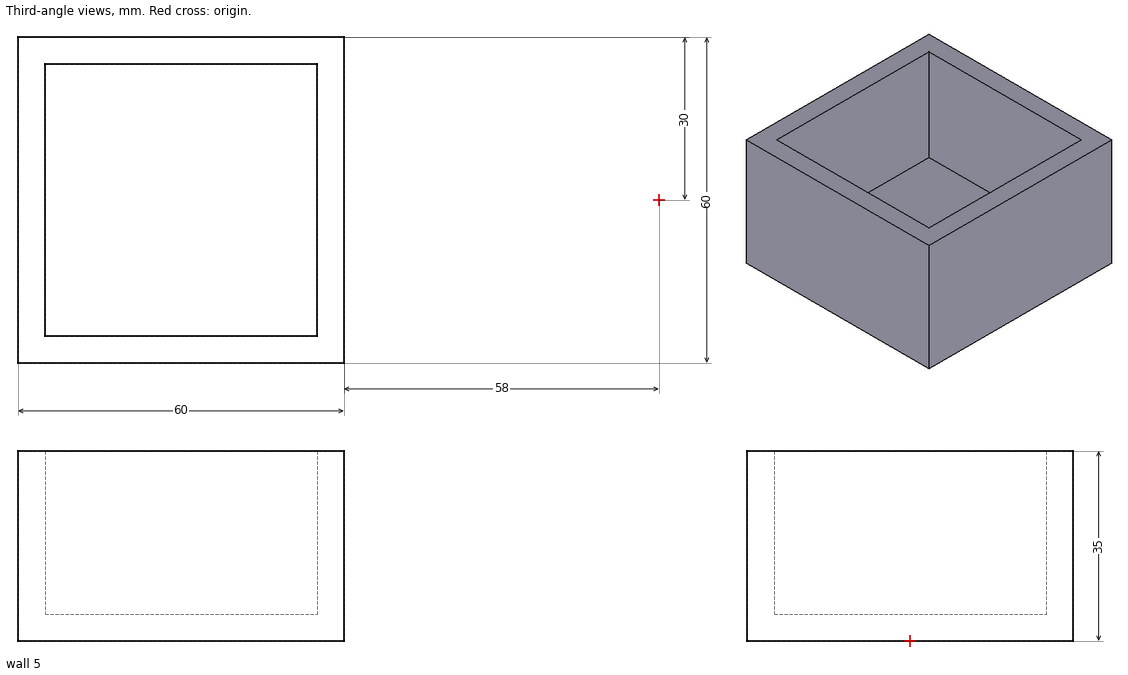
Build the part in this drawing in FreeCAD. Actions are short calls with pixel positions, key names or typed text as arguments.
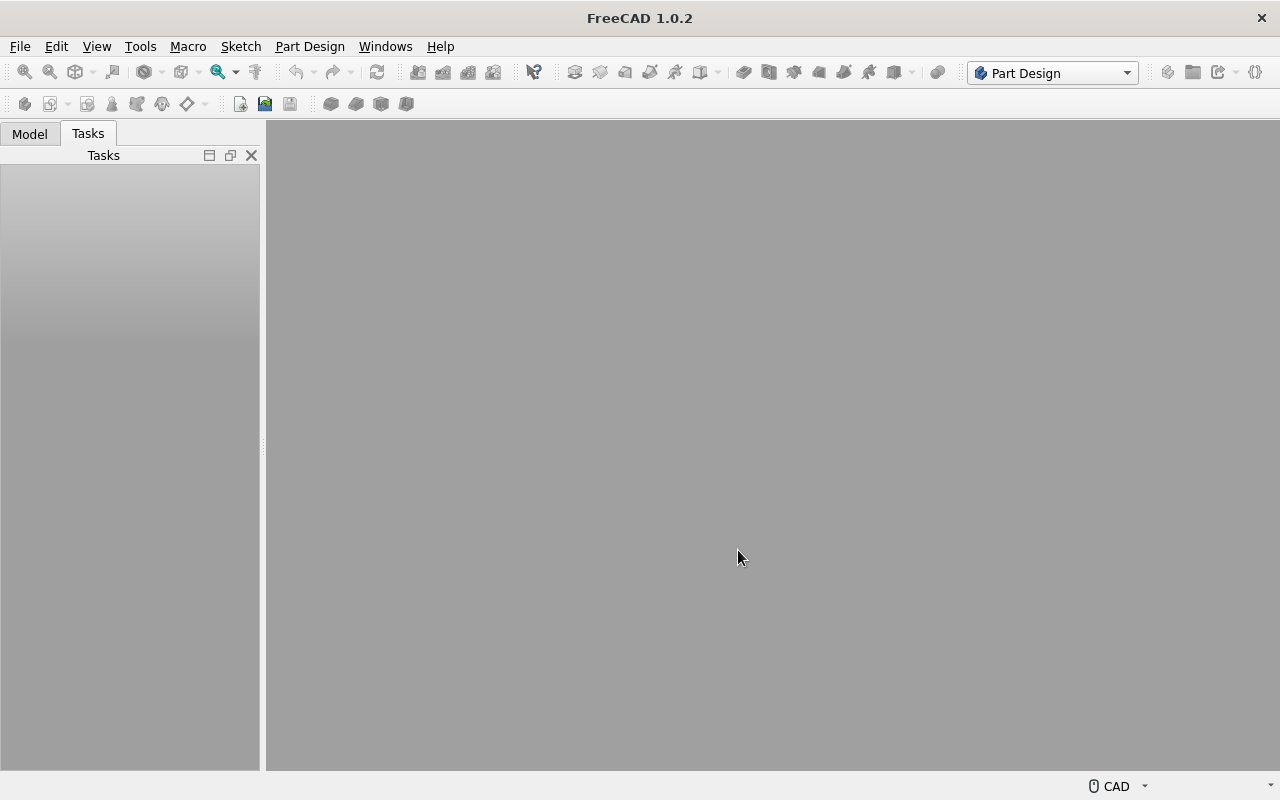
key(ctrl+n)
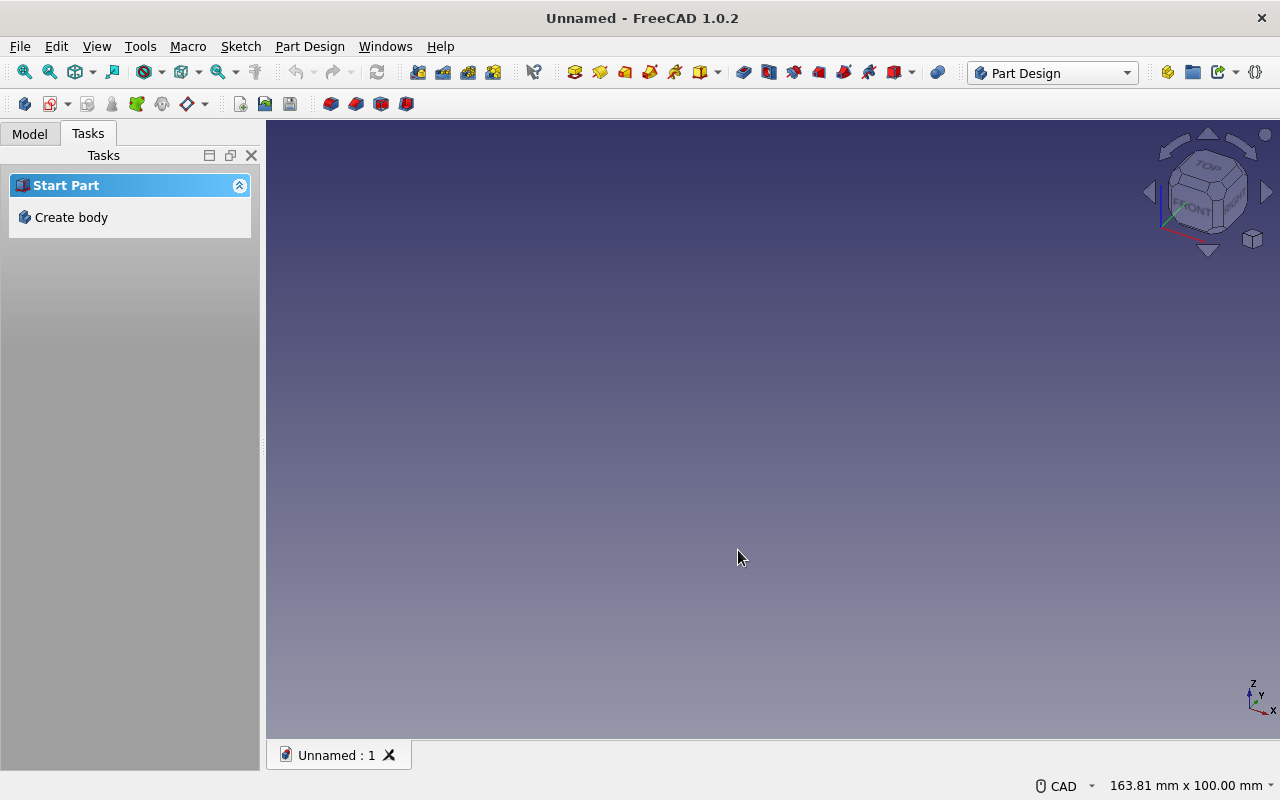
click(50, 104)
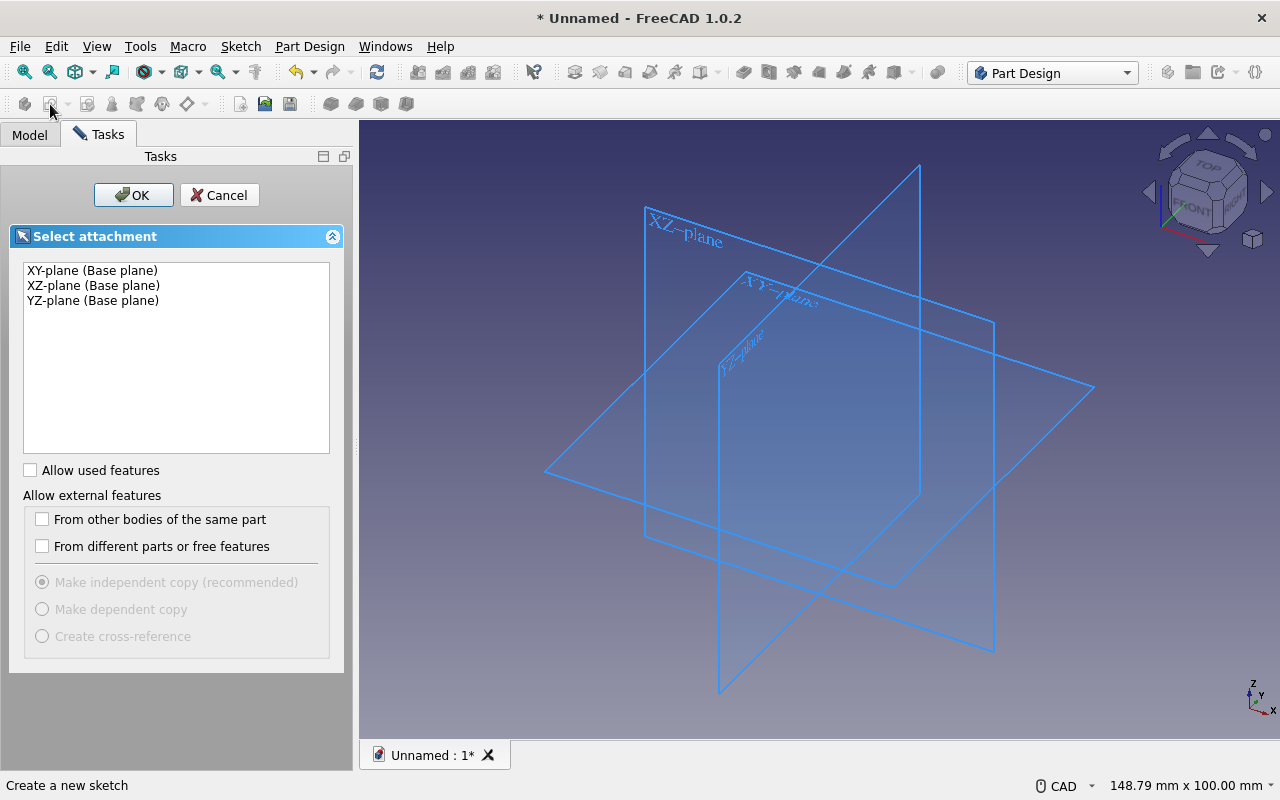
click(84, 270)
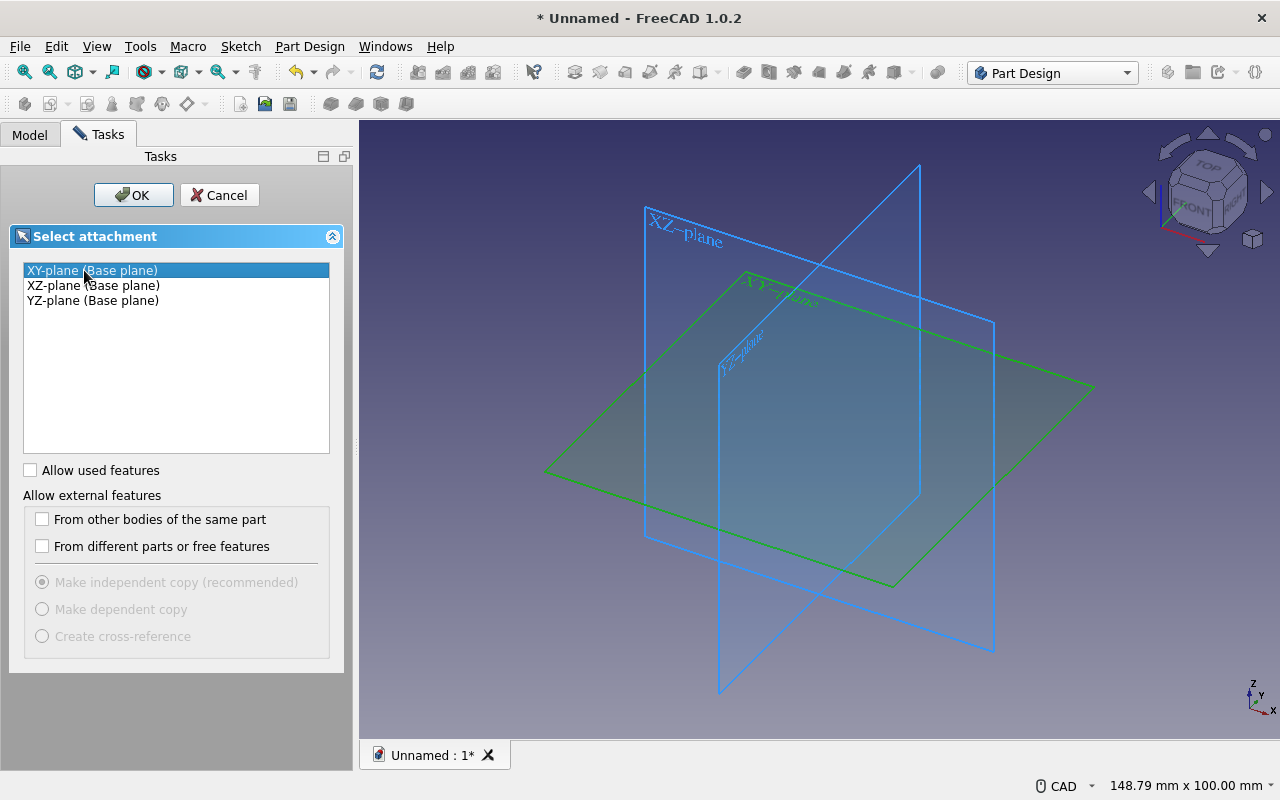
click(134, 195)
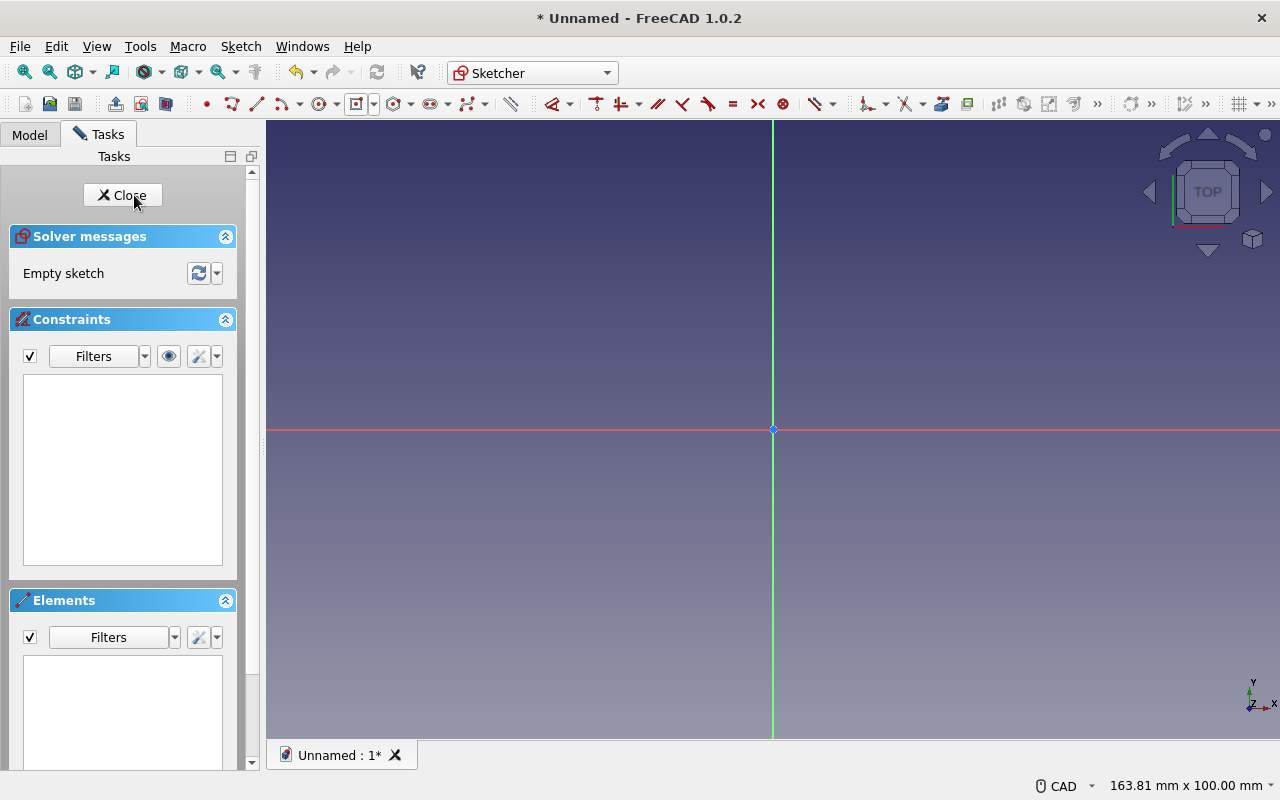
scroll(1115, 429, down, 2)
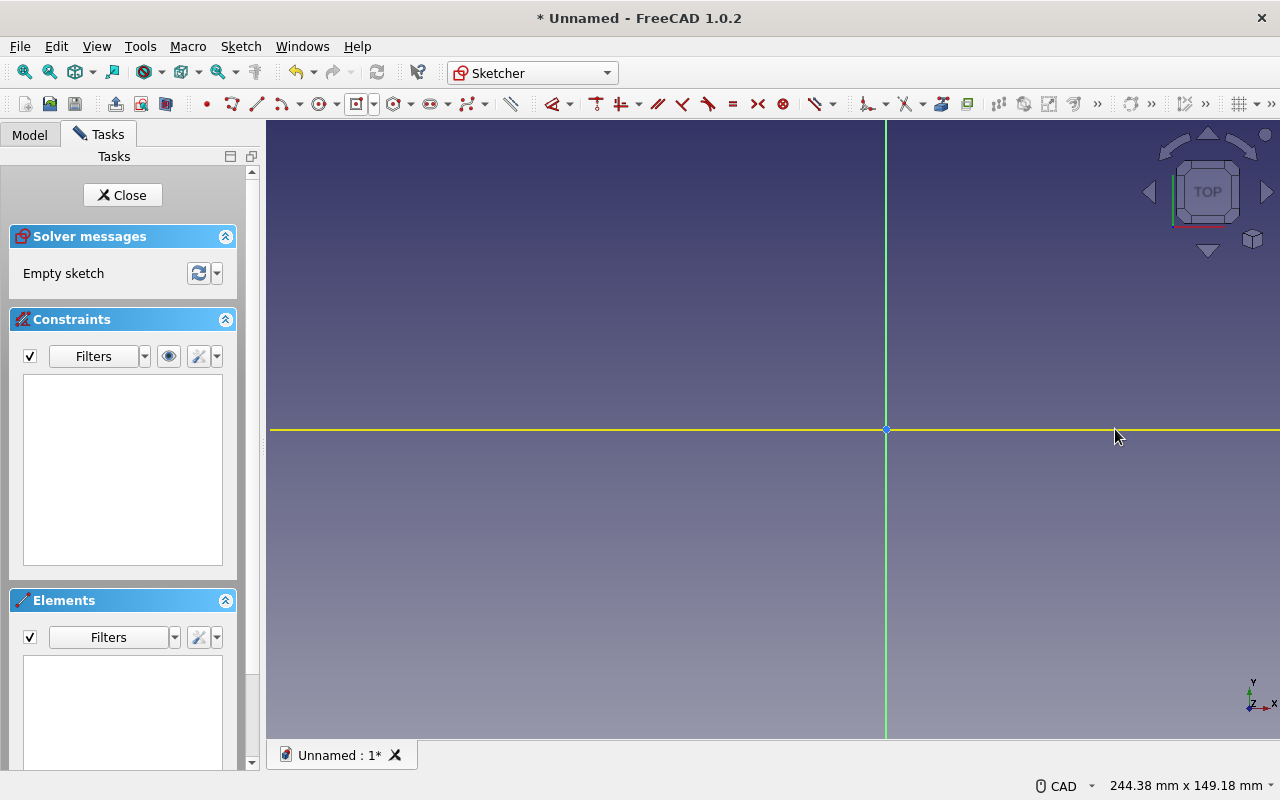
key(g)
key(r)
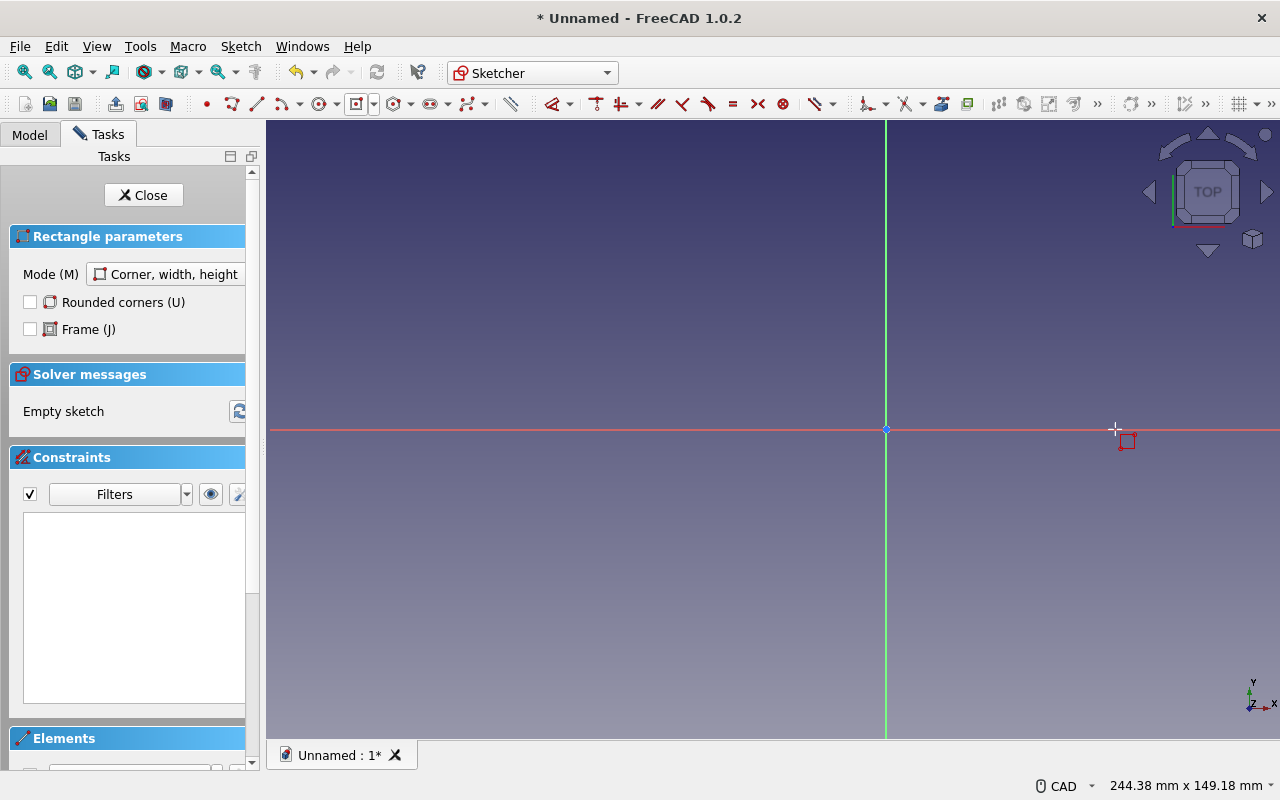
click(396, 305)
move(645, 554)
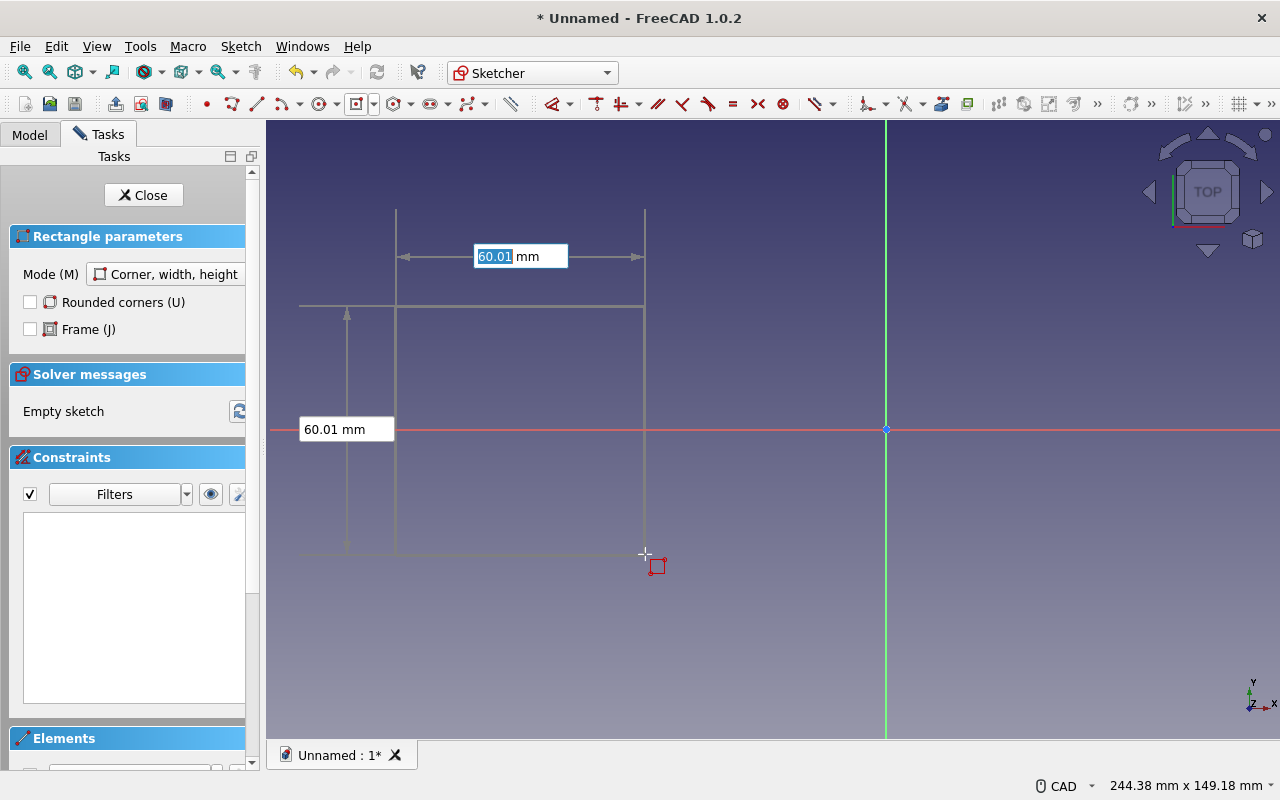
text(60)
key(Tab)
text(60)
key(Return)
key(Escape)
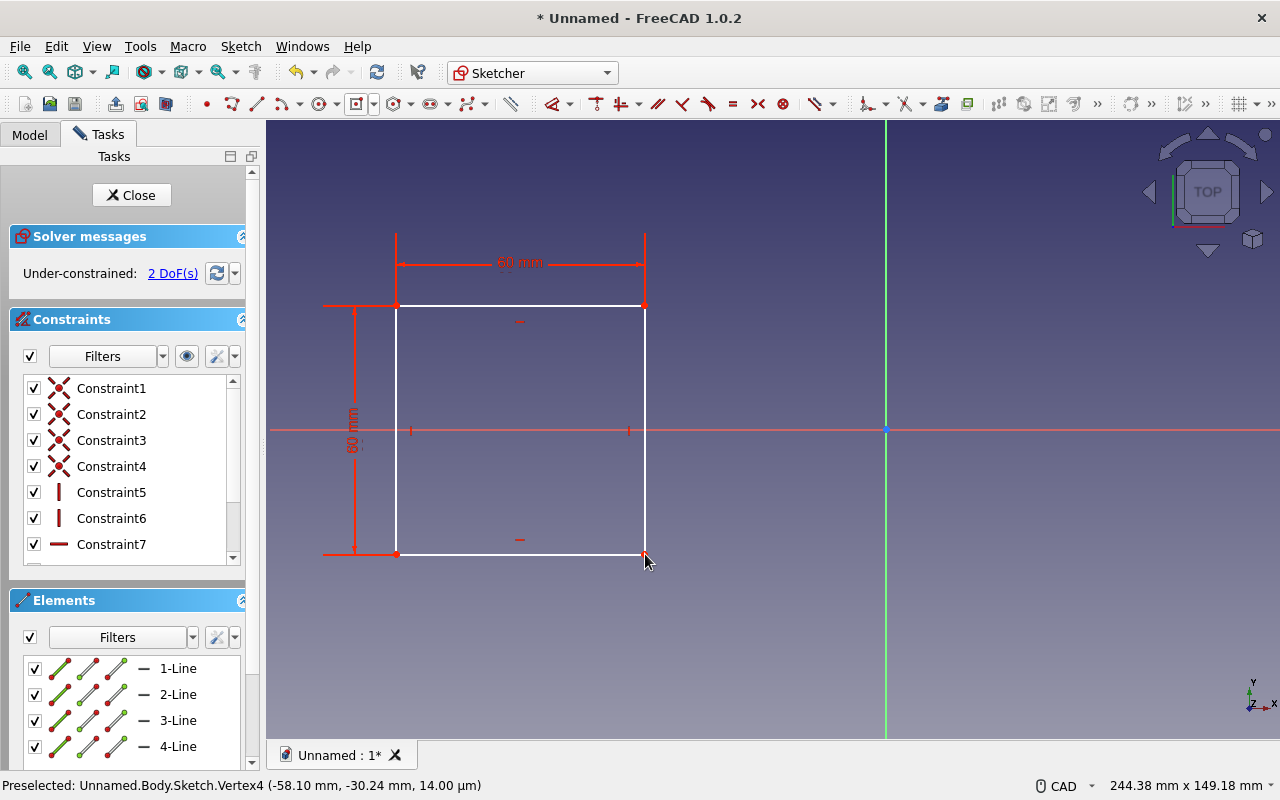
key(d)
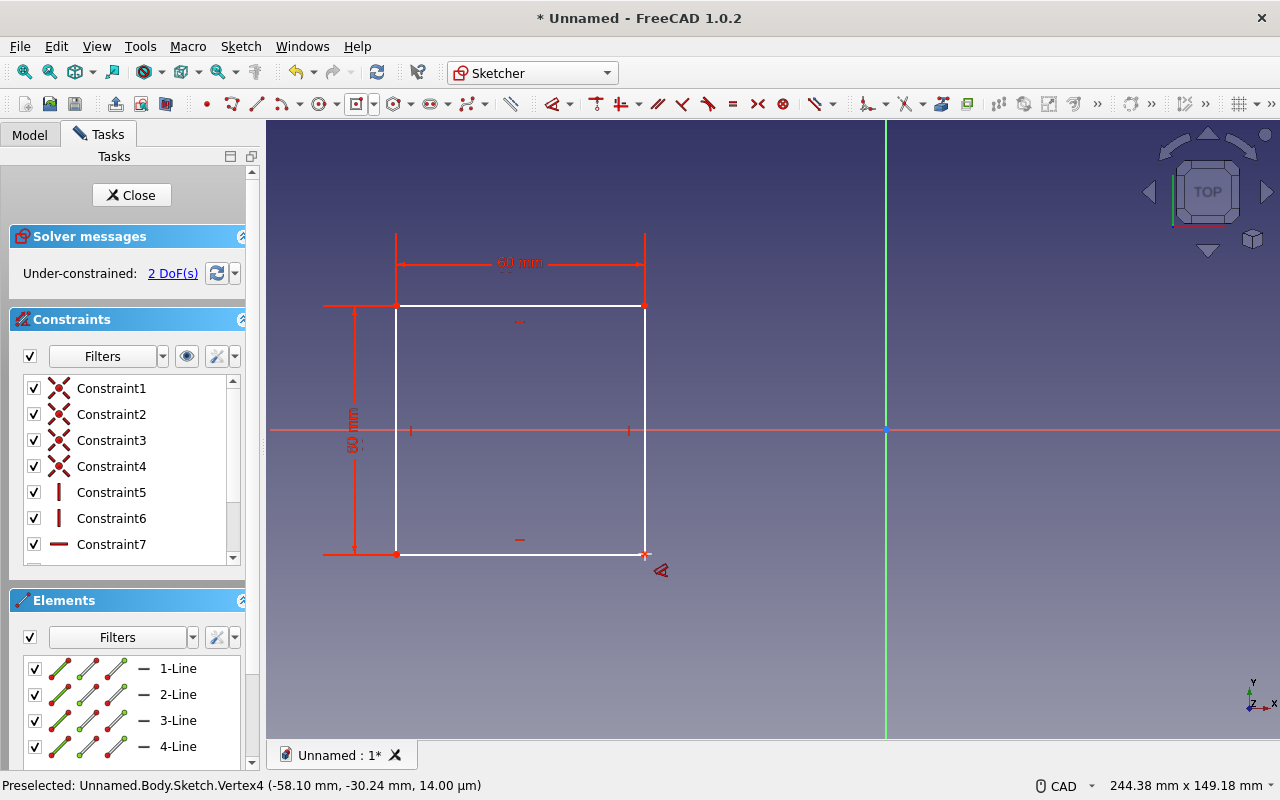
click(396, 306)
click(362, 368)